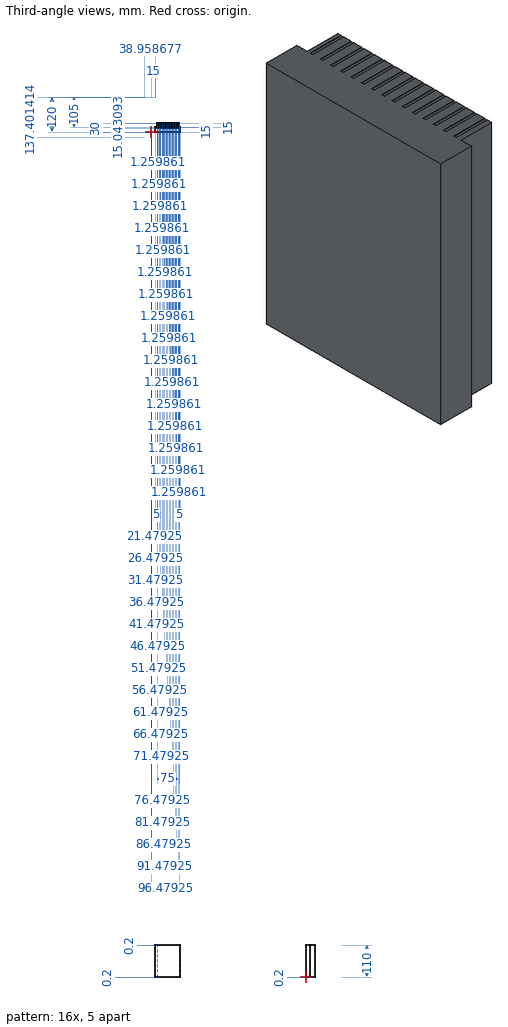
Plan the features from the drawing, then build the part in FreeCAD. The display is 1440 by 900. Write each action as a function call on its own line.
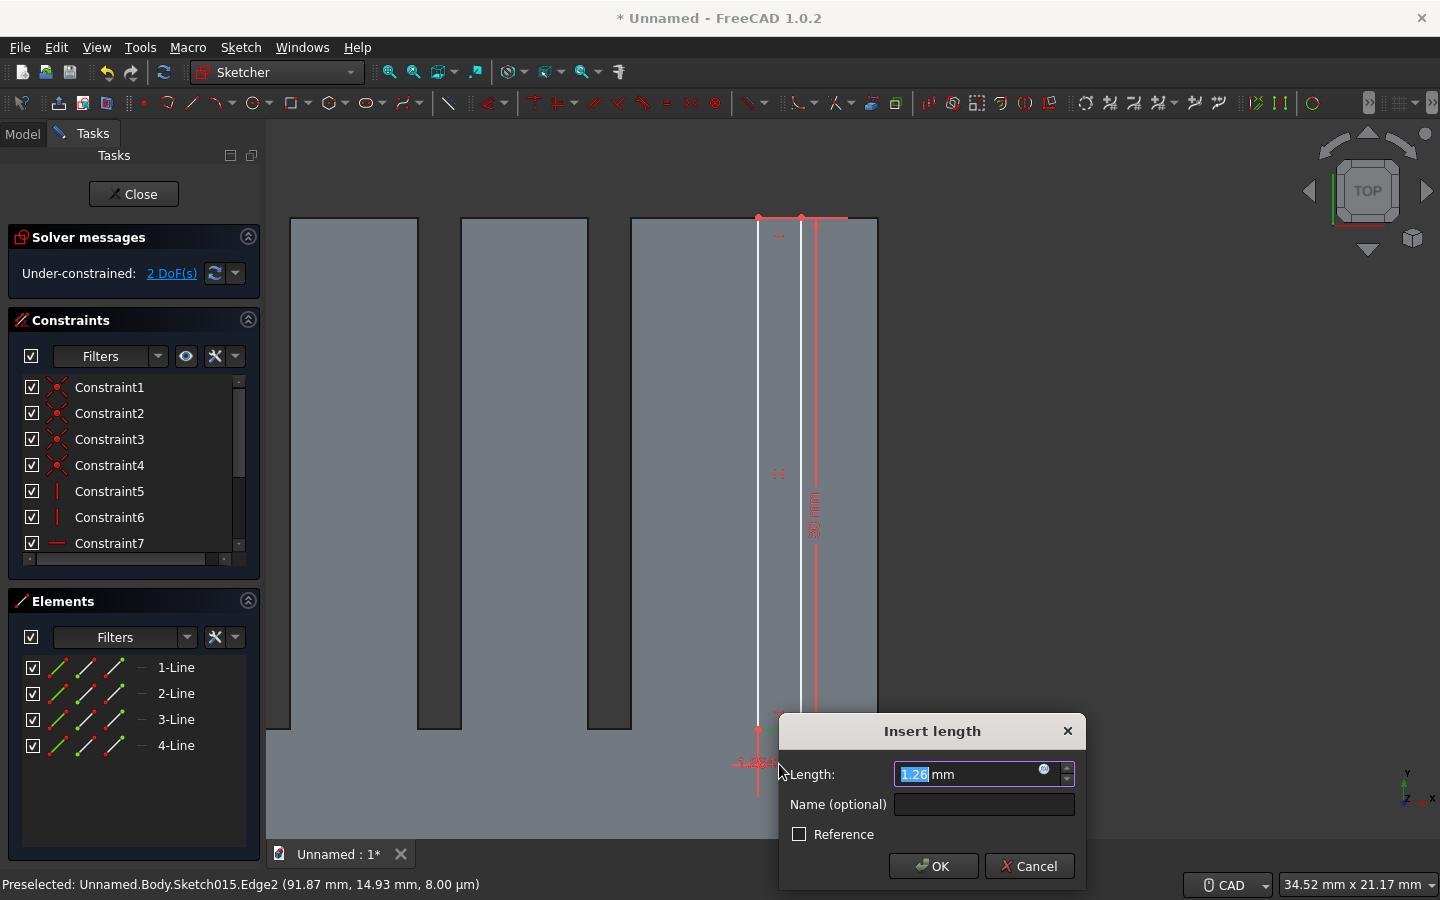
text(1.259861)
key(Return)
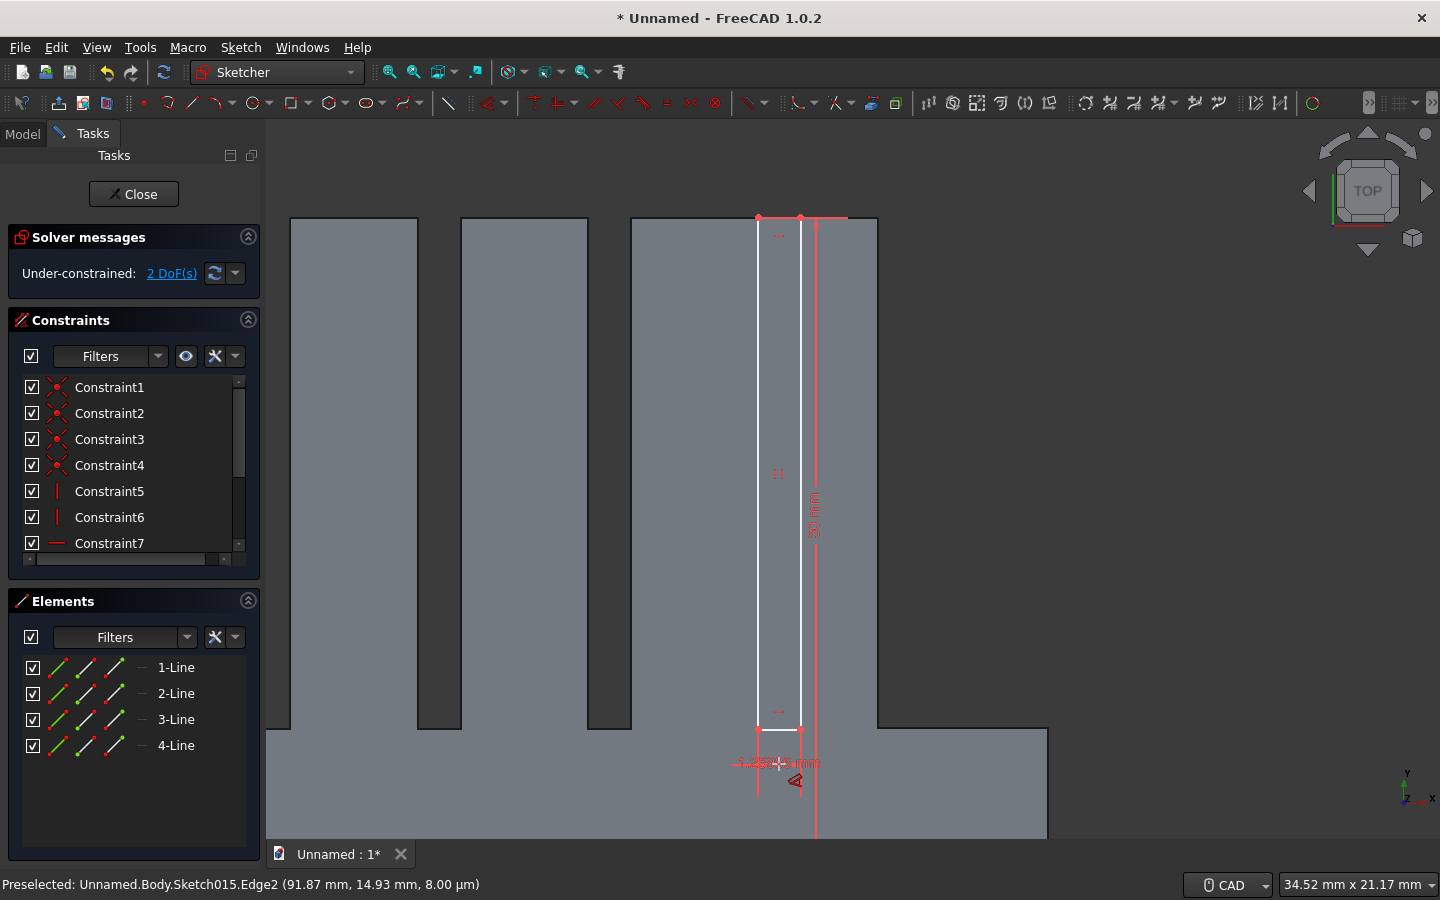
click(758, 371)
click(724, 474)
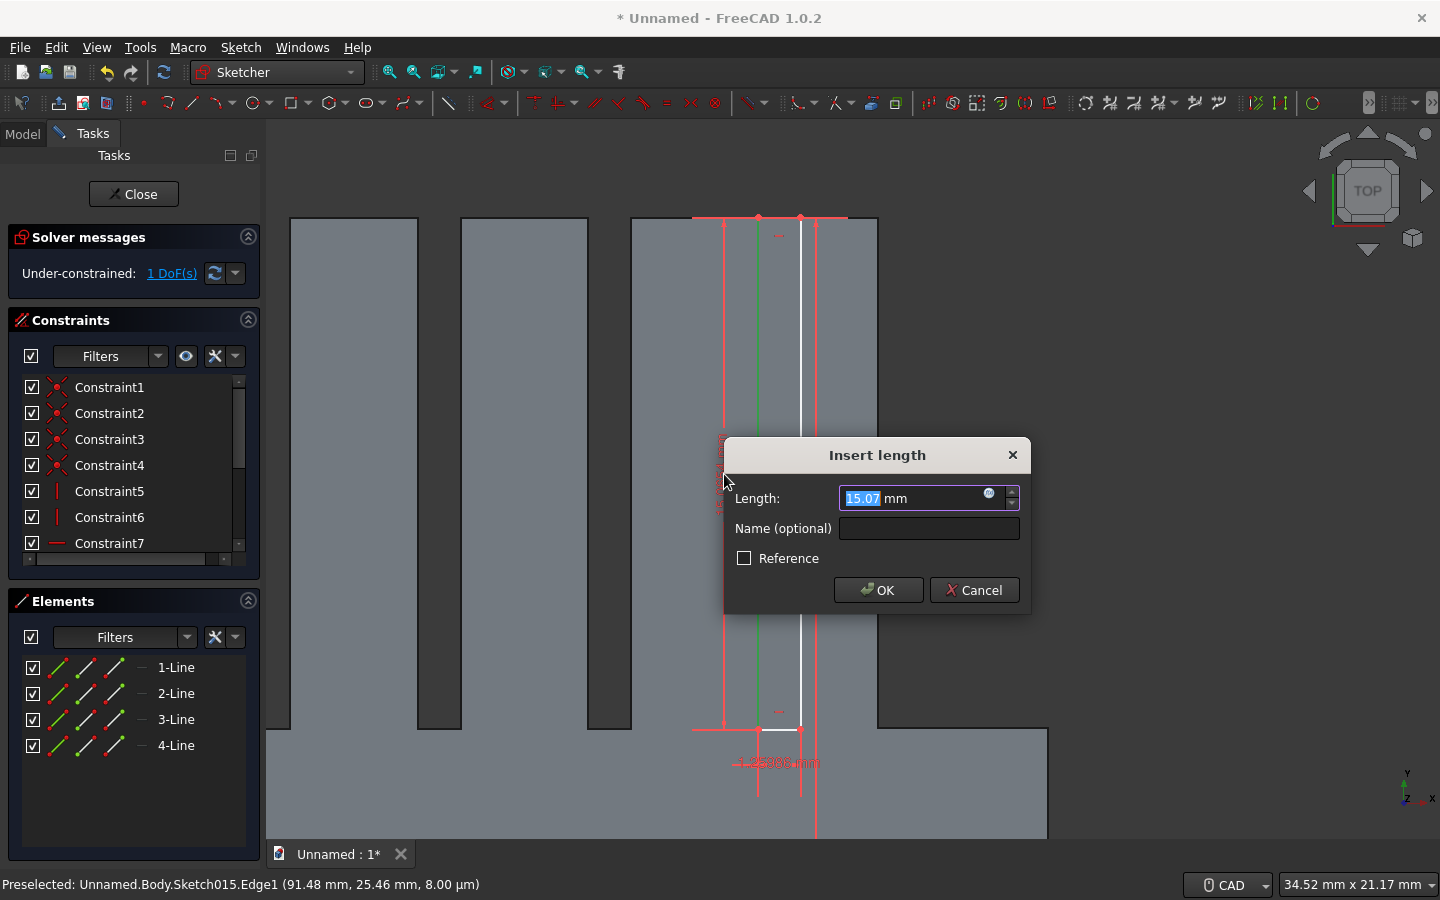
text(15.043093)
key(Return)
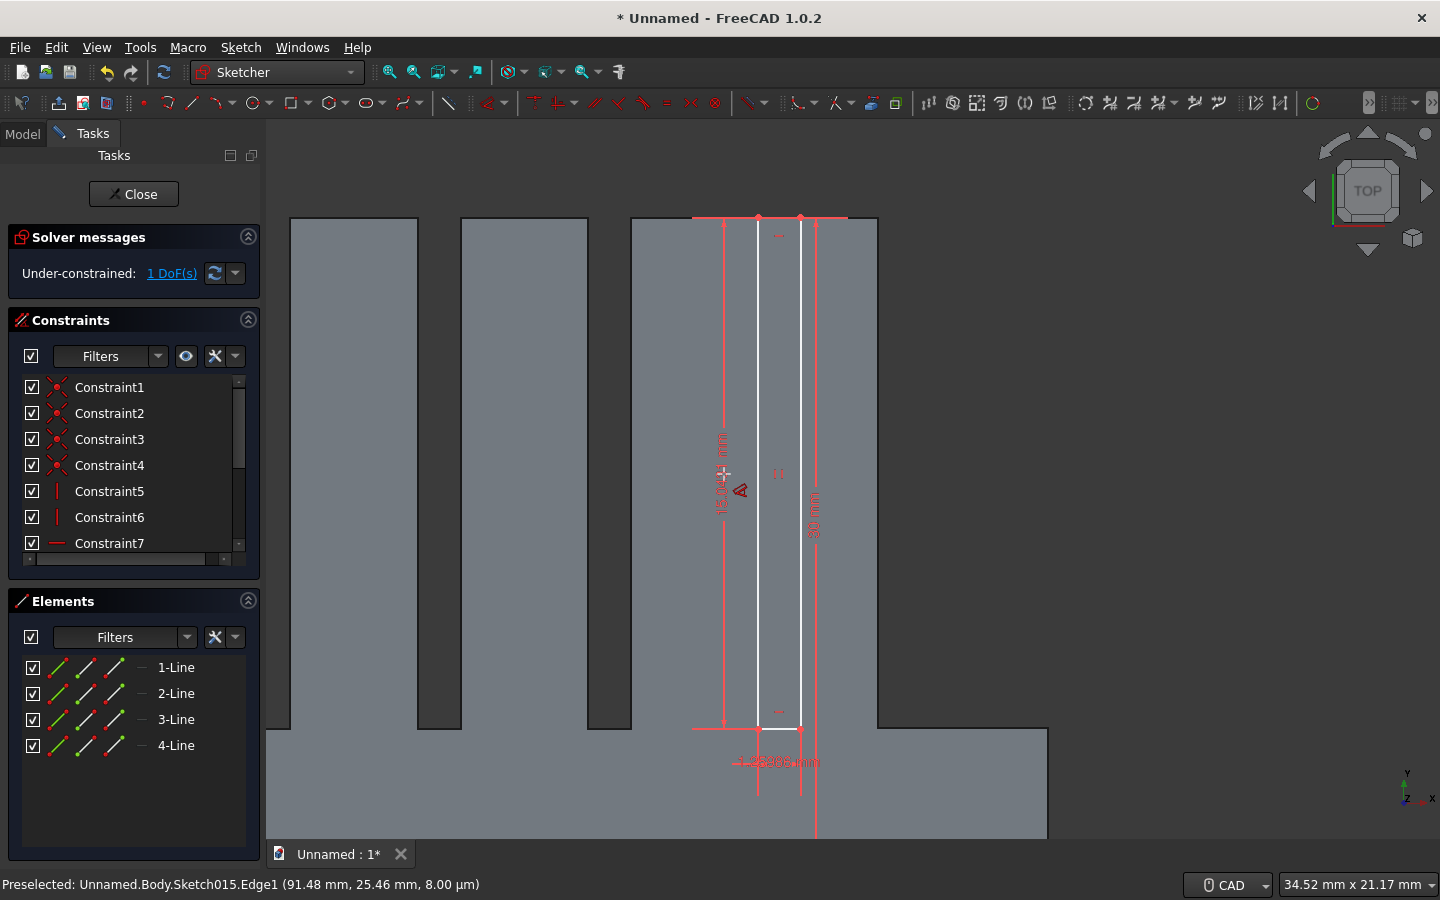
click(758, 218)
click(526, 184)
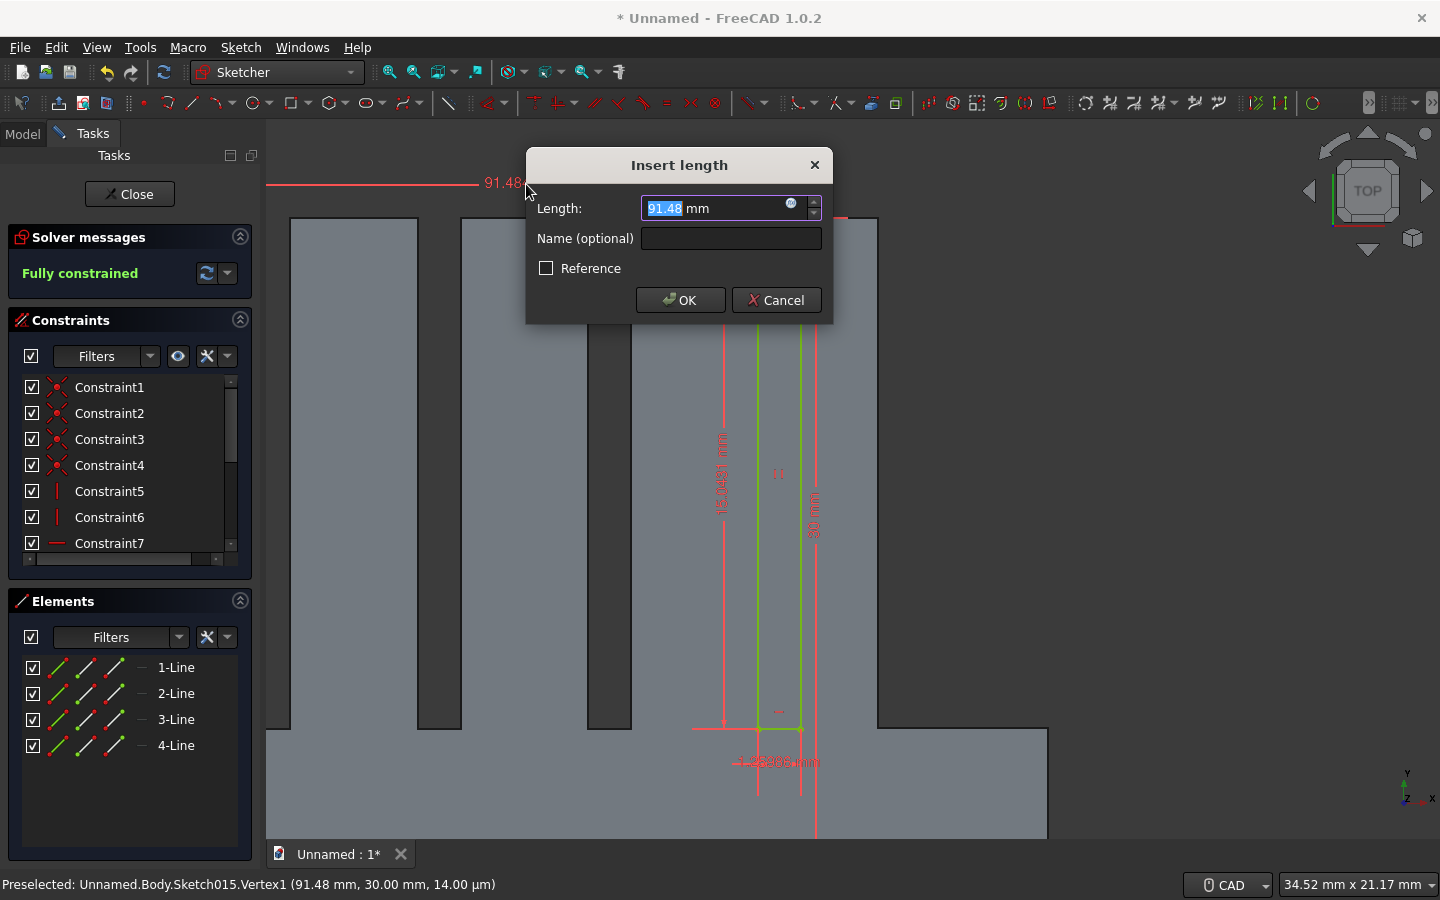
text(91.47925)
key(Return)
key(Escape)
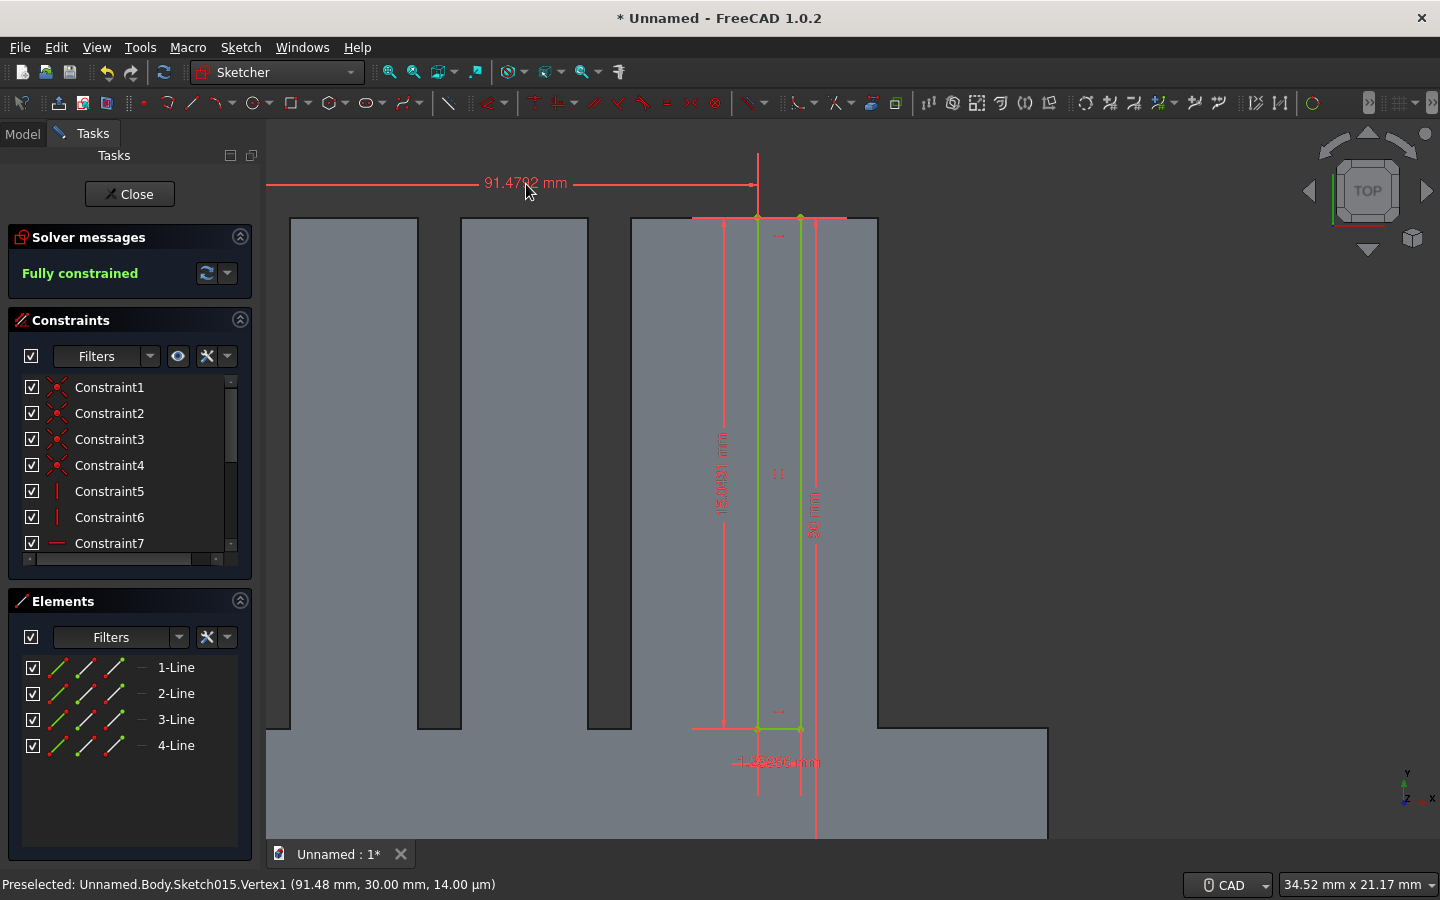
click(130, 194)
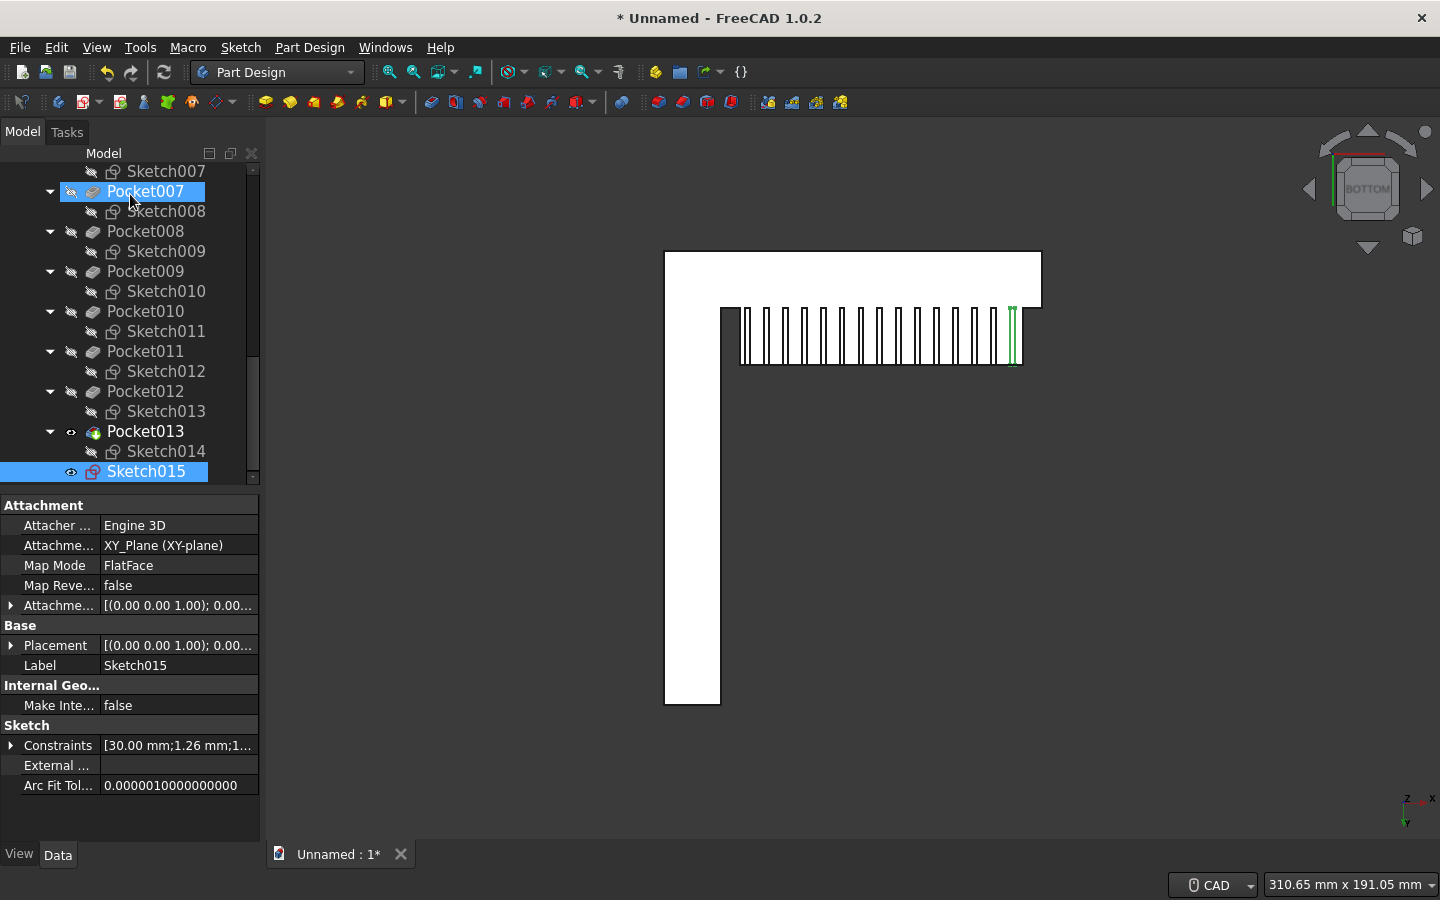
click(432, 102)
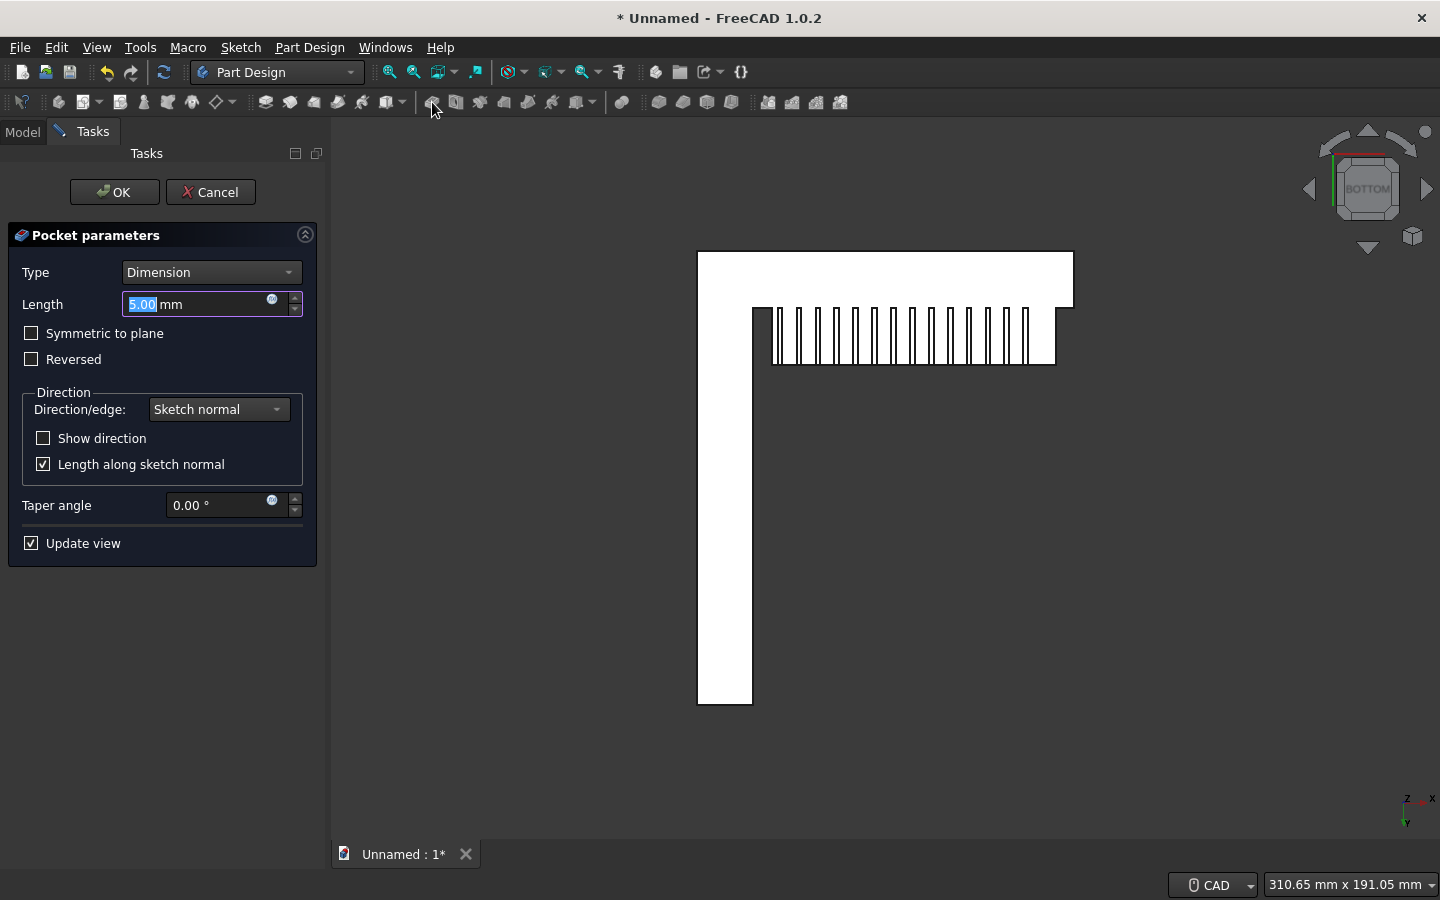
text(0.2)
key(Tab)